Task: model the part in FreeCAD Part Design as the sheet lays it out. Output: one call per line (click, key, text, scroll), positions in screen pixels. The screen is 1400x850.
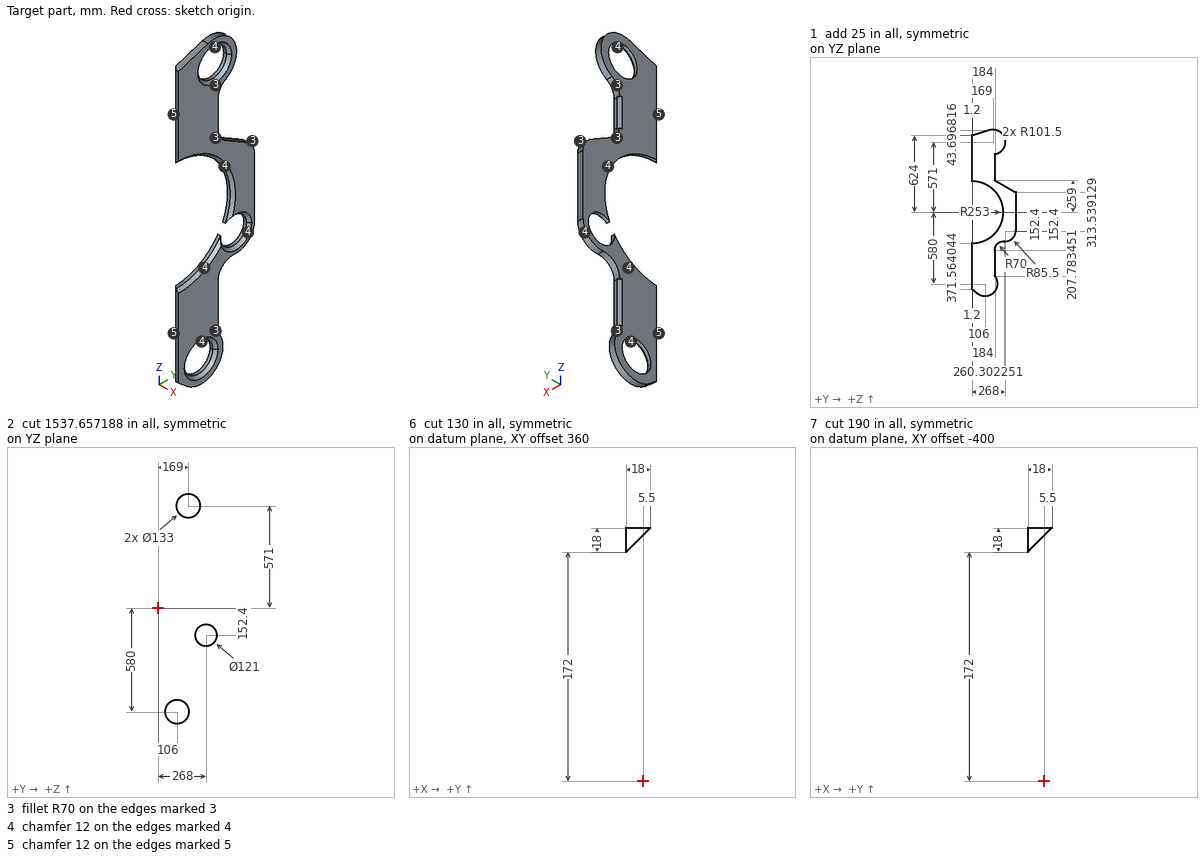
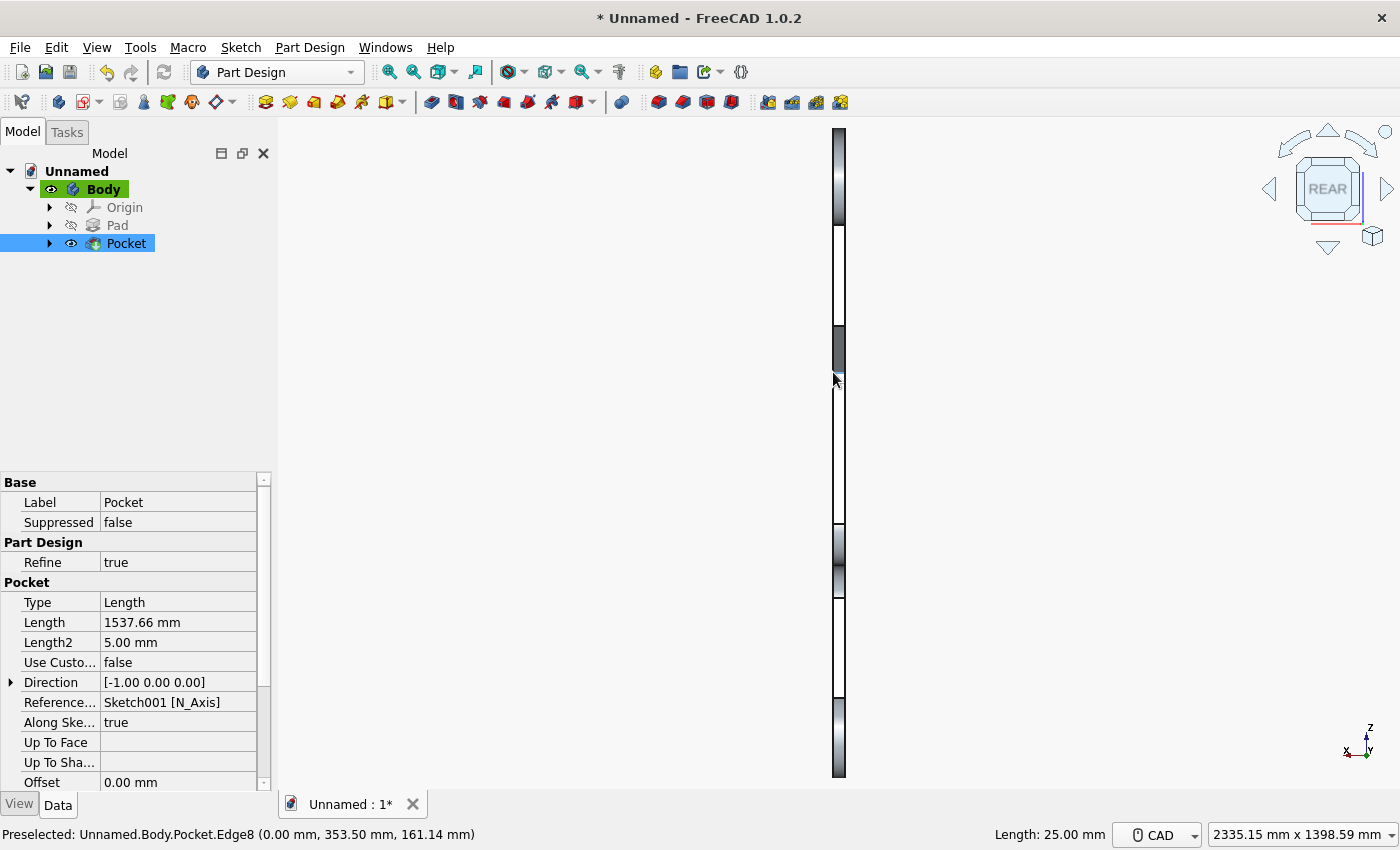
scroll(839, 224, up, 7)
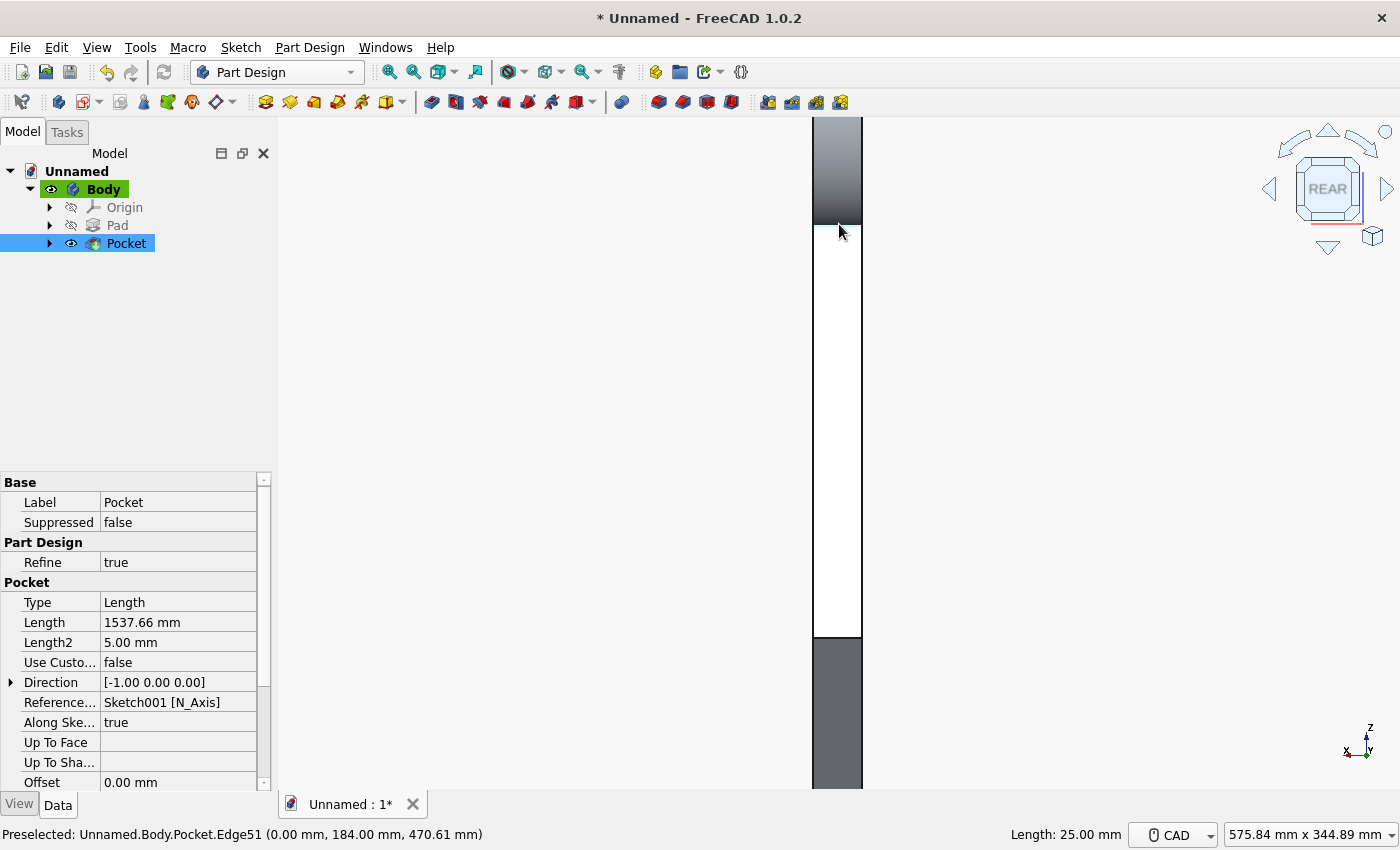
key(v)
key(f)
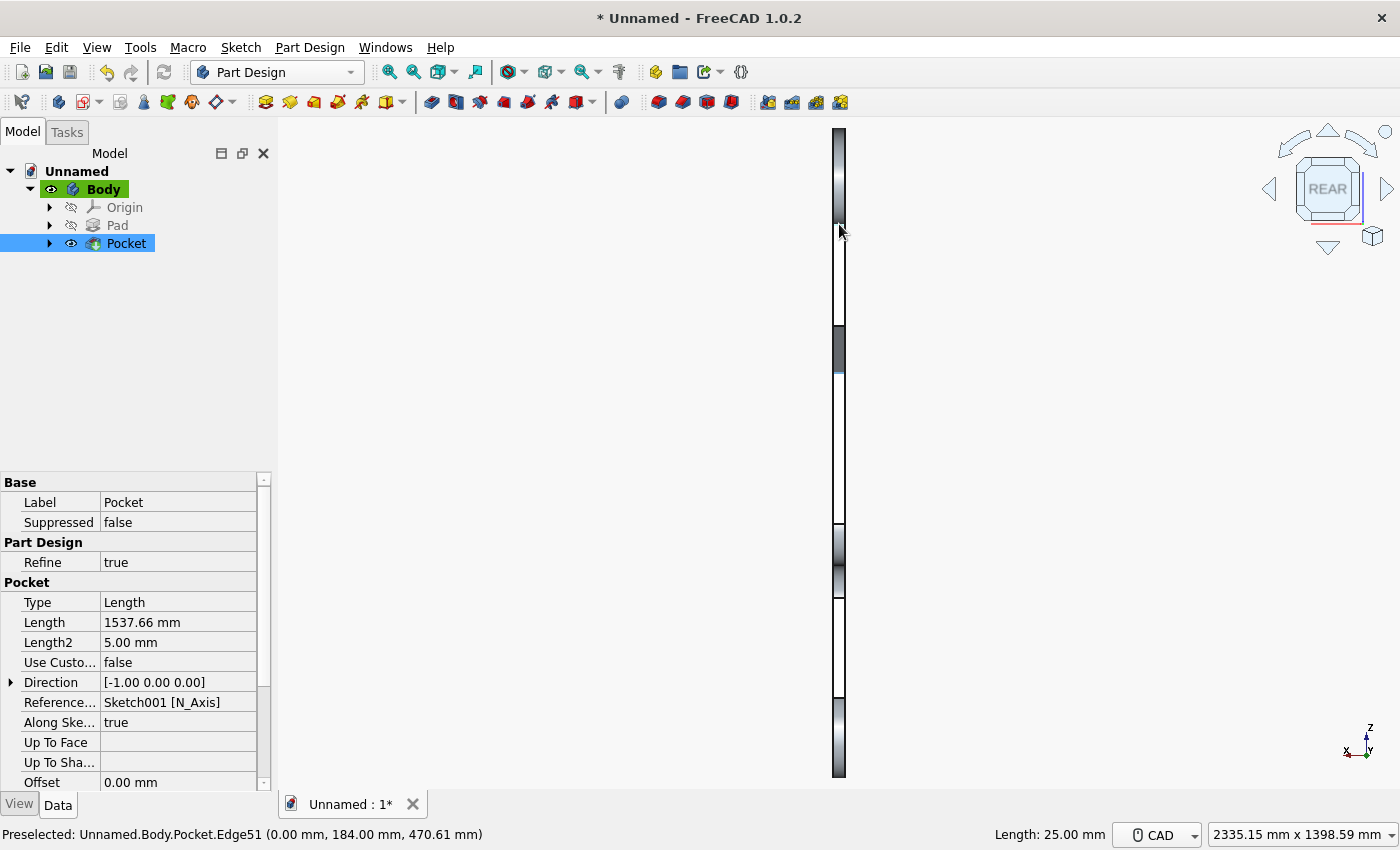
key(6)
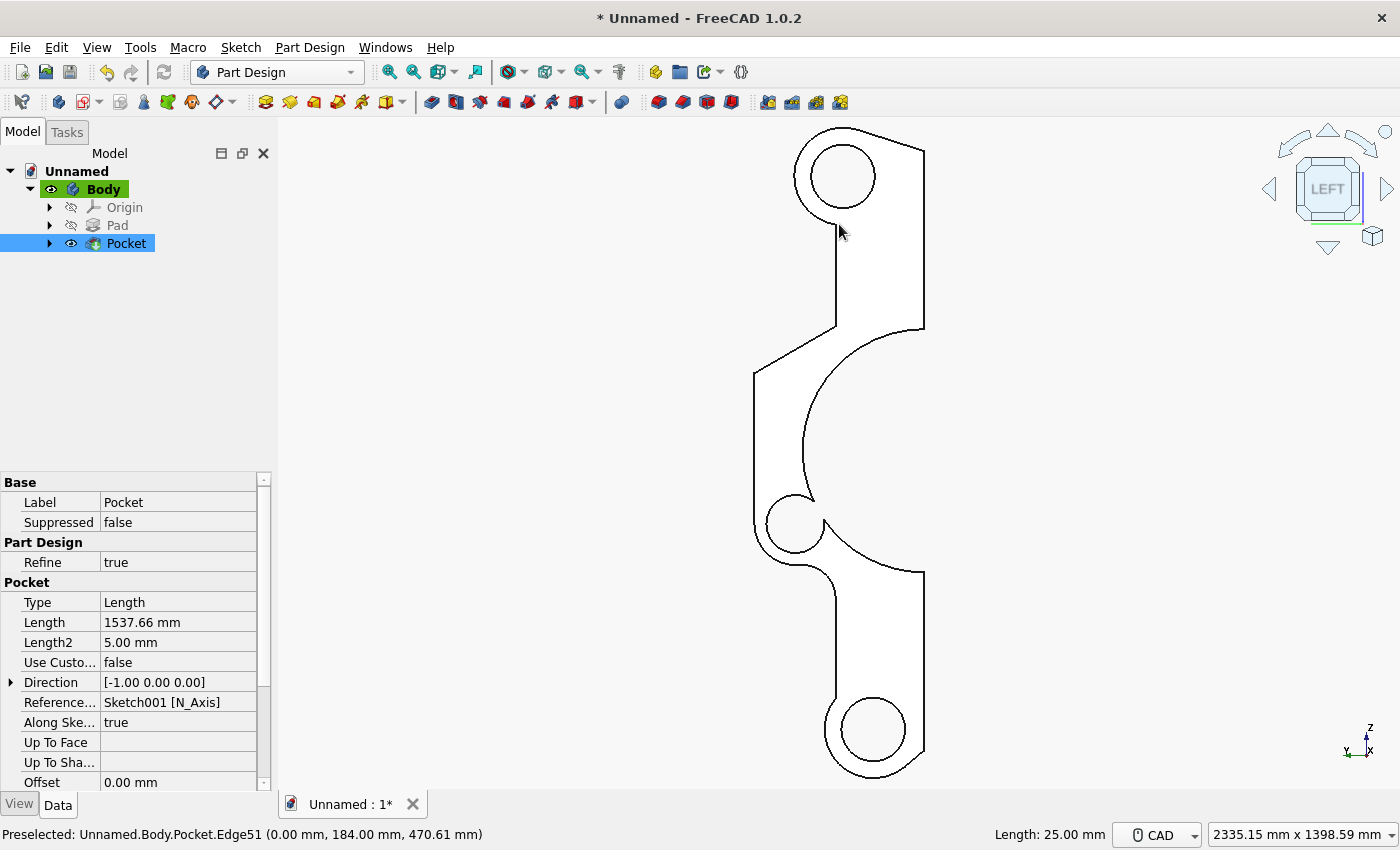
scroll(836, 224, up, 7)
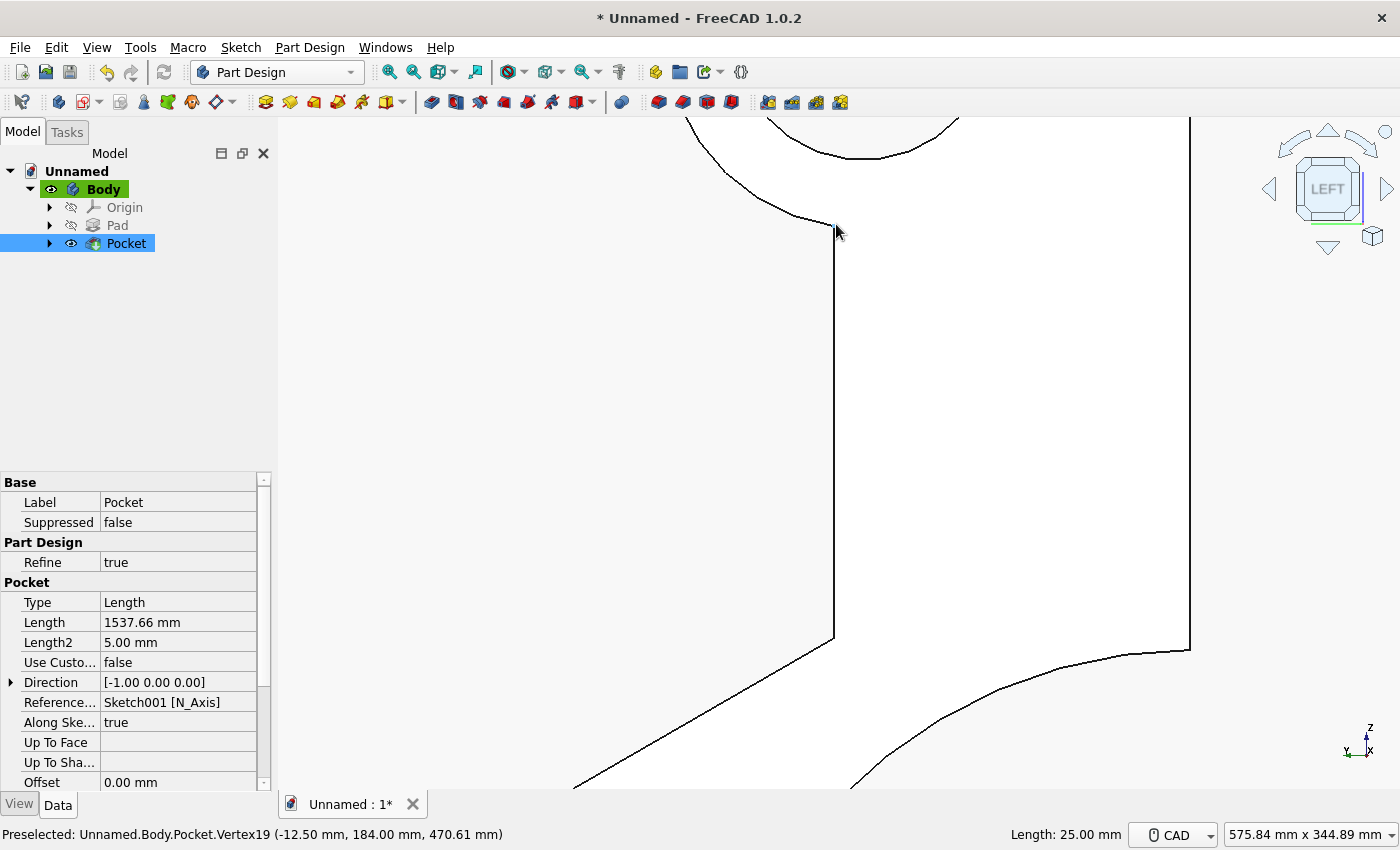
click(390, 72)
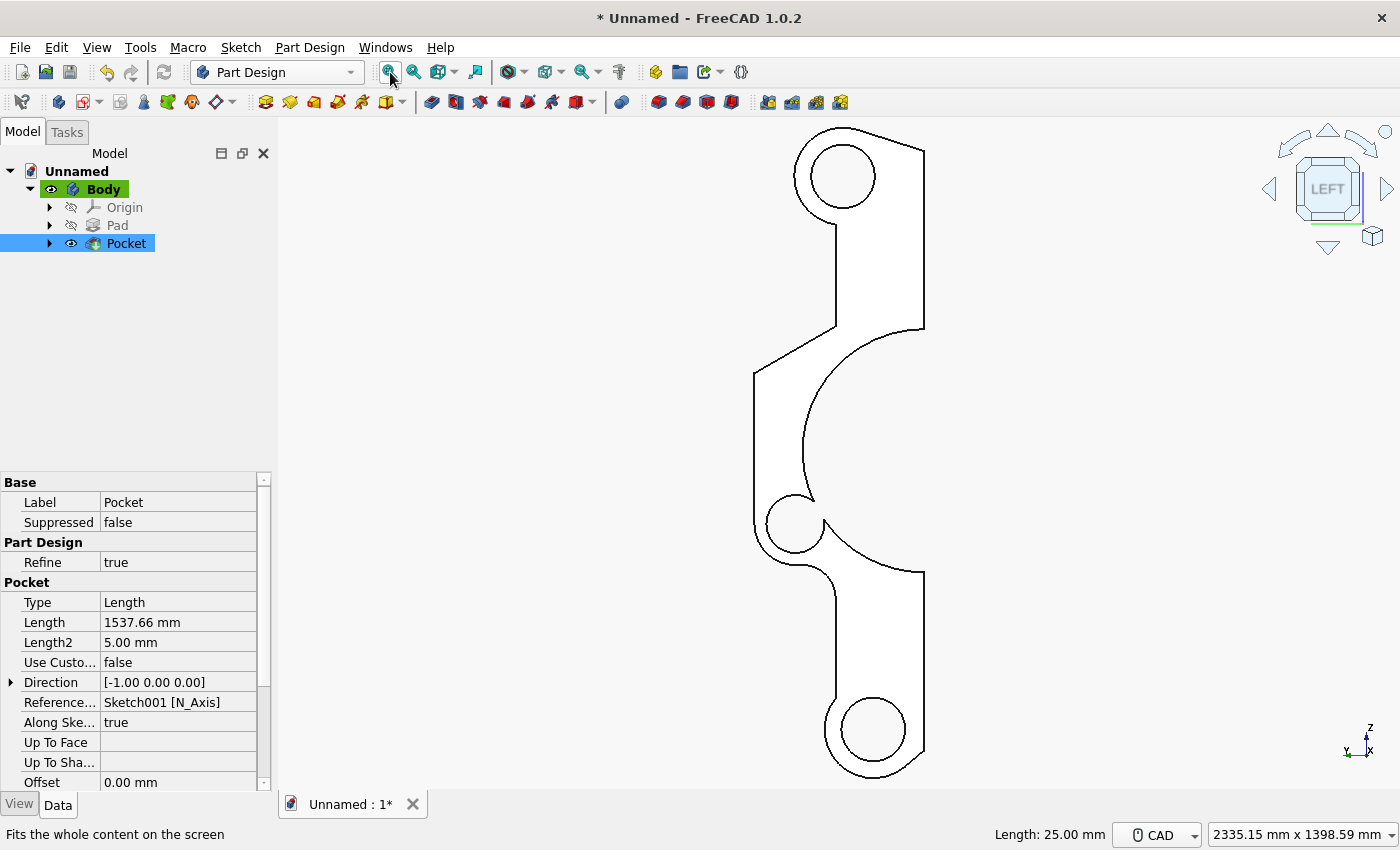
key(v)
key(3)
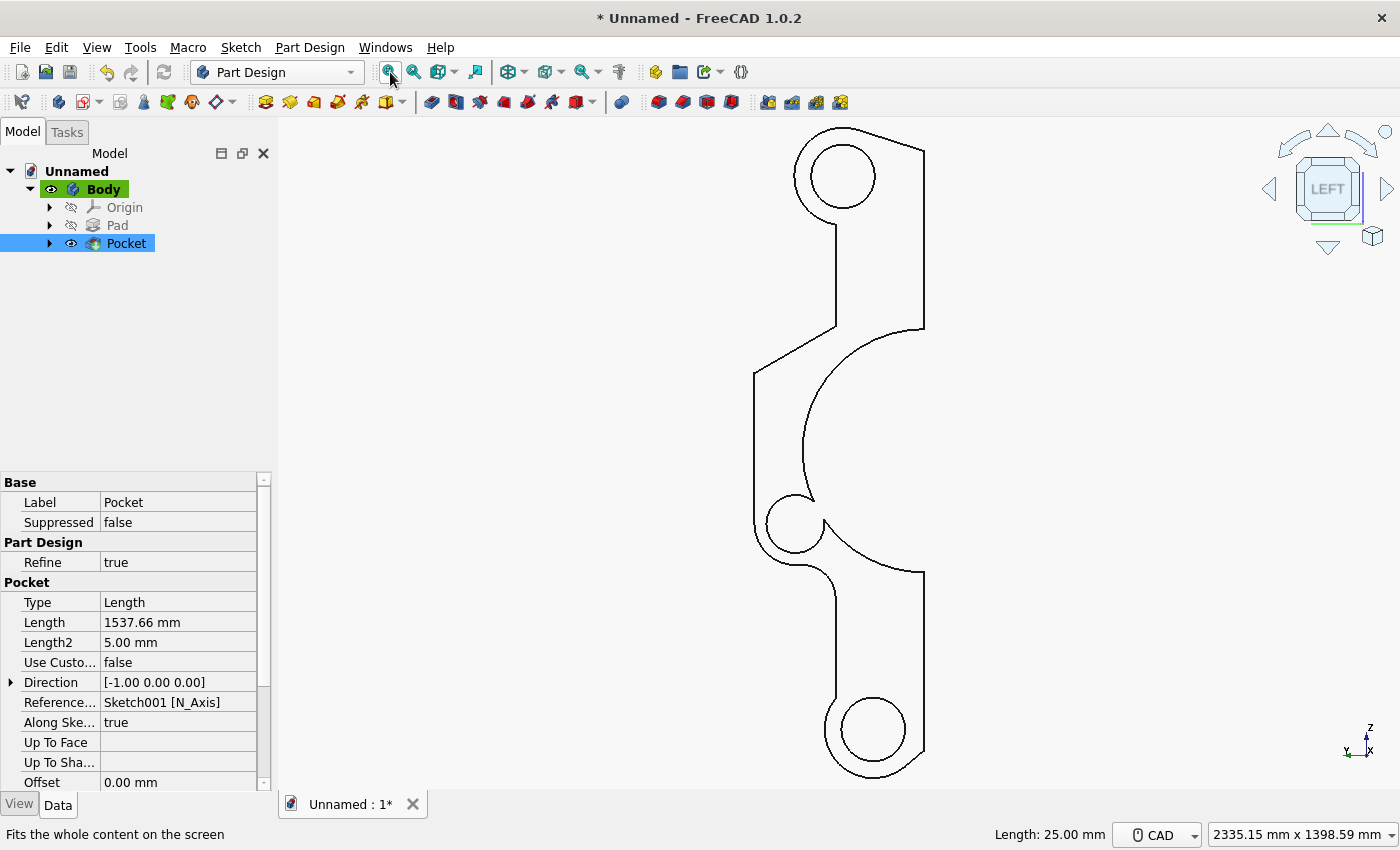
key(0)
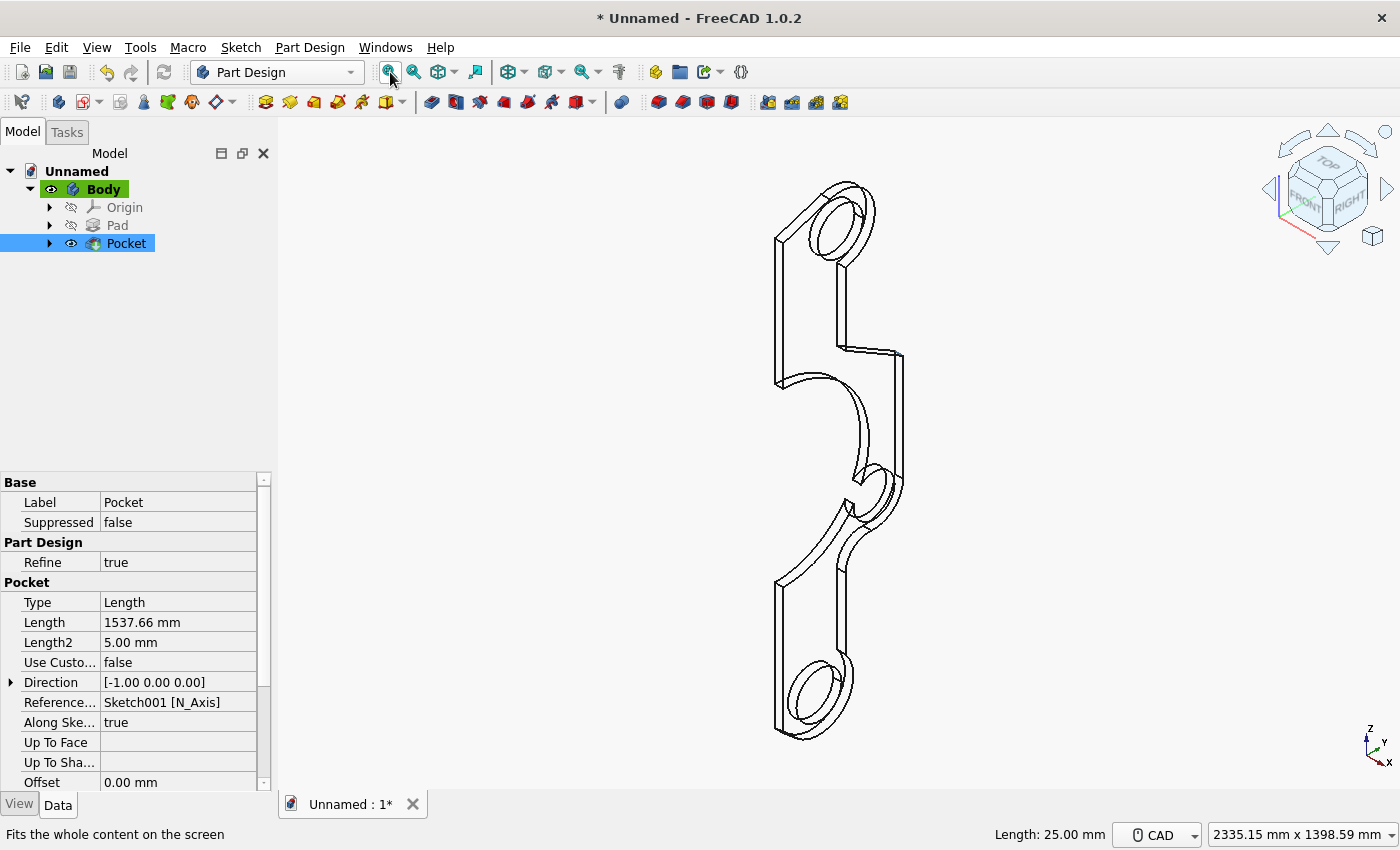
click(839, 346, ctrl)